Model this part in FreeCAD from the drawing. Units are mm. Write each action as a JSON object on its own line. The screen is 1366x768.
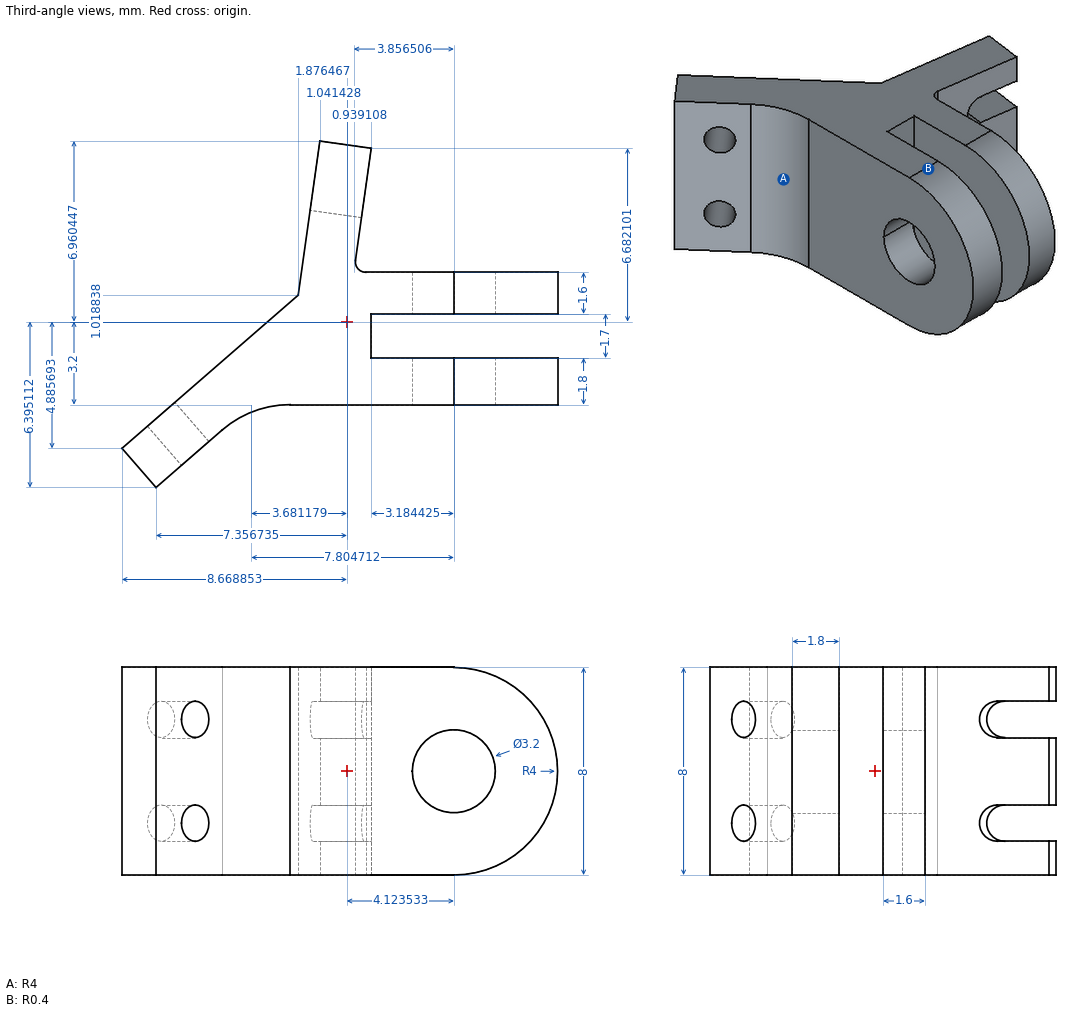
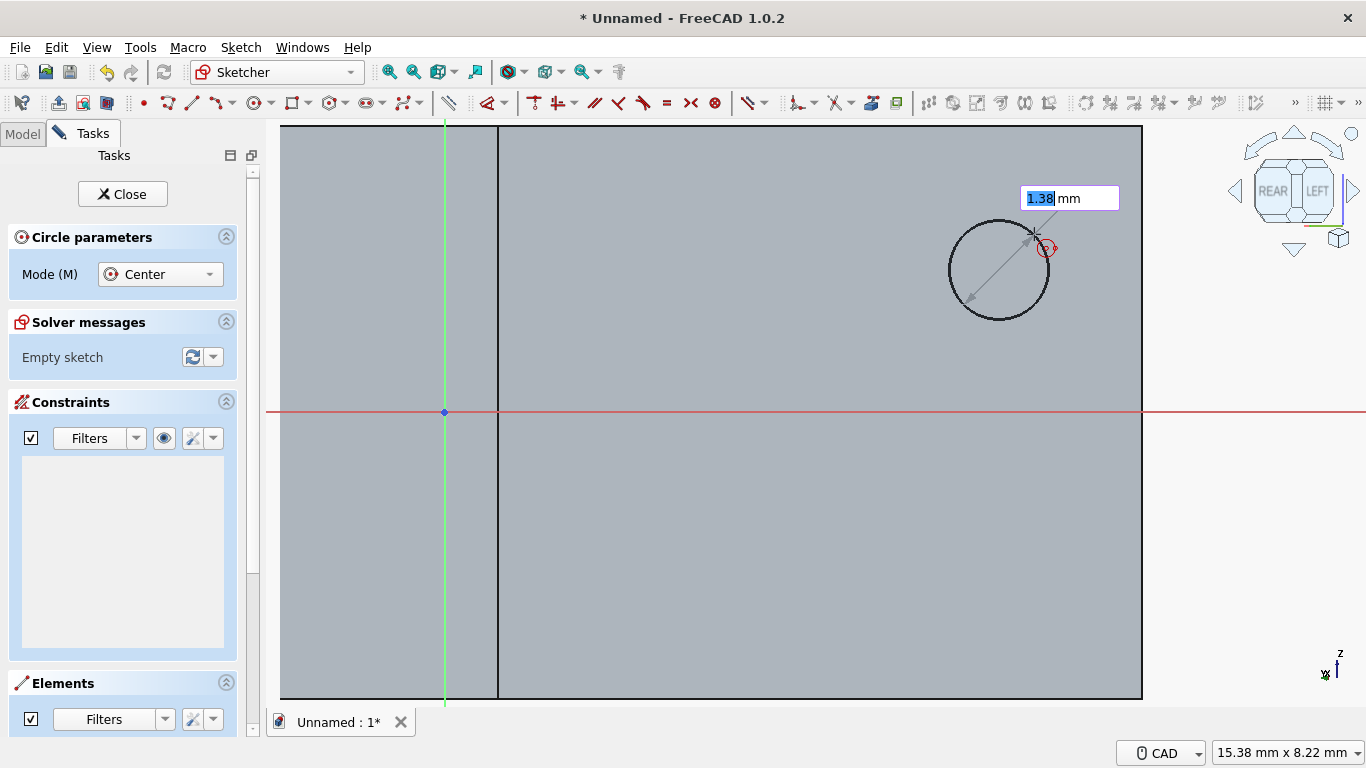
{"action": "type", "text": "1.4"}
{"action": "key", "text": "Return"}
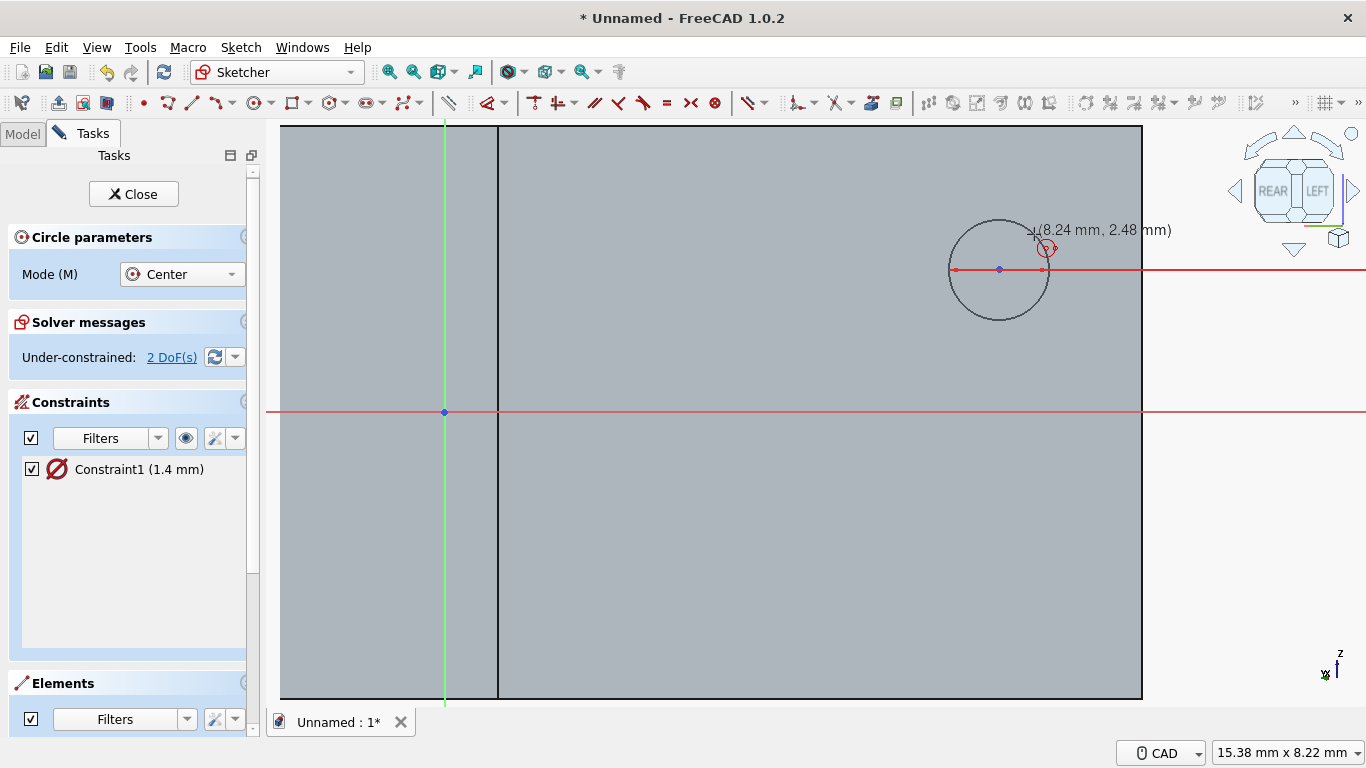
{"action": "left_click", "coordinate": [999, 555]}
{"action": "mouse_move", "coordinate": [1034, 520]}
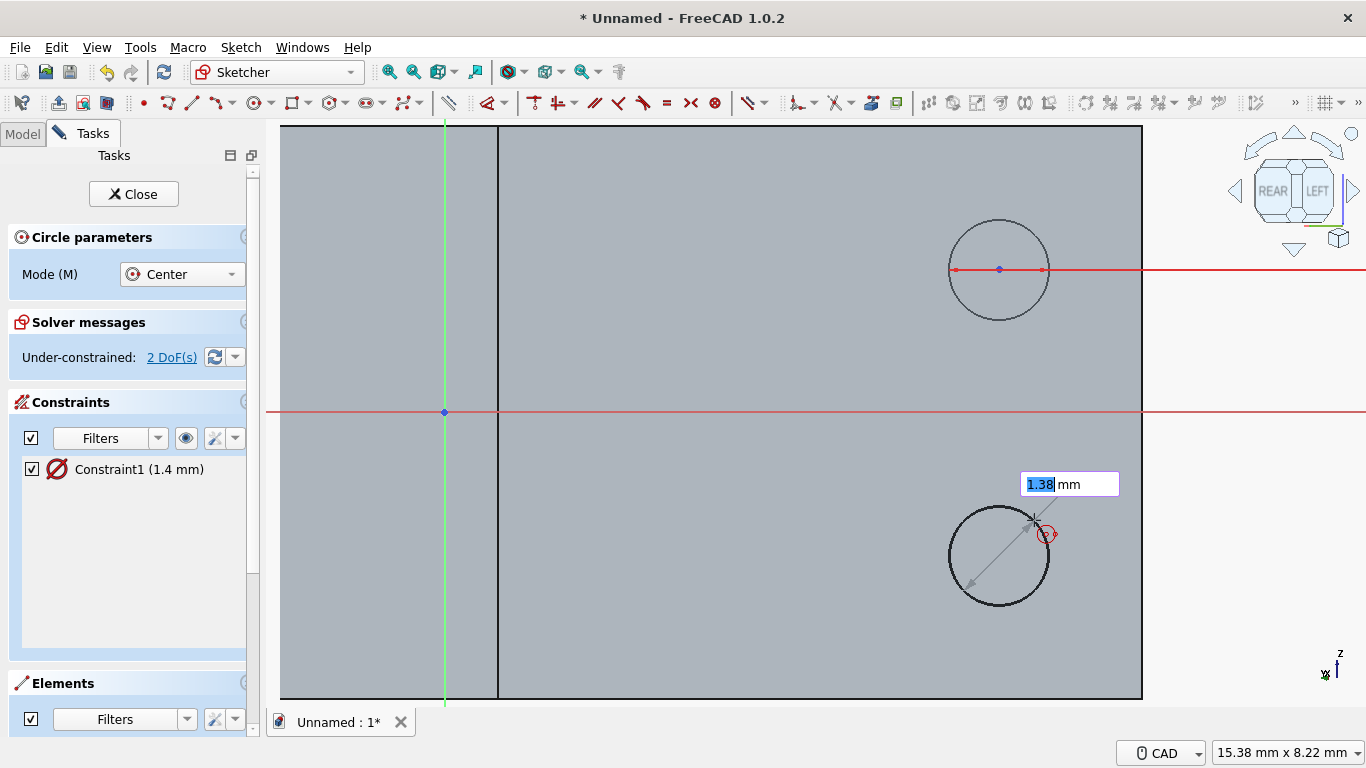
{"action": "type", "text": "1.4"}
{"action": "key", "text": "Return"}
{"action": "key", "text": "Escape"}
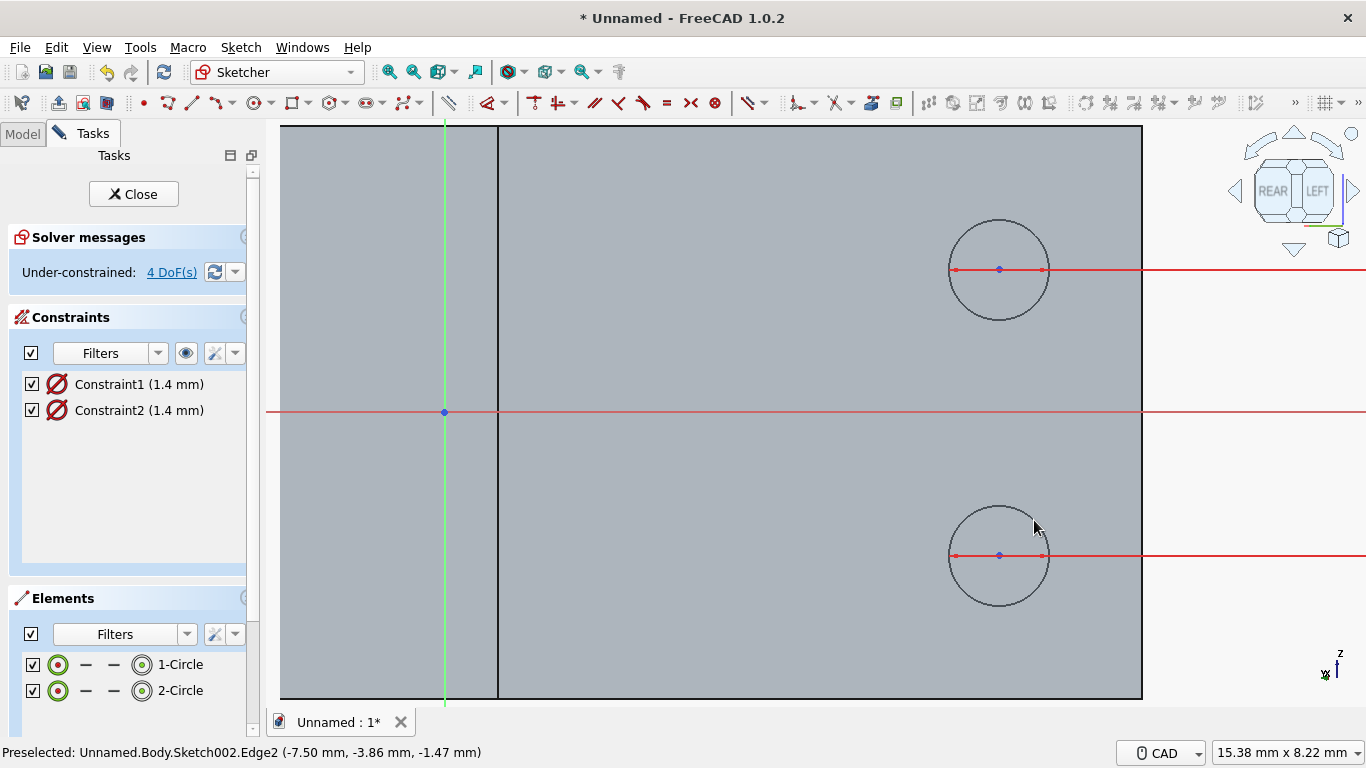
{"action": "left_click", "coordinate": [999, 270]}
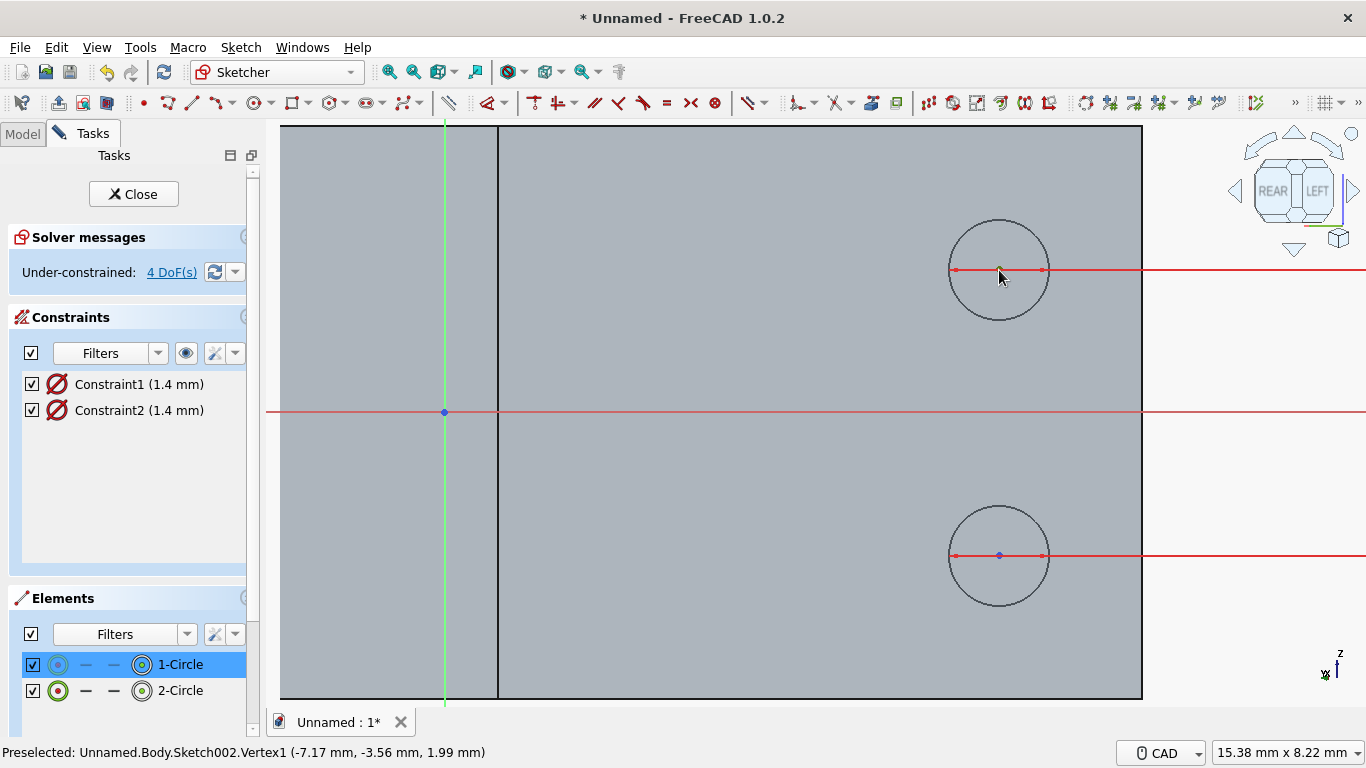
{"action": "left_click", "coordinate": [999, 556]}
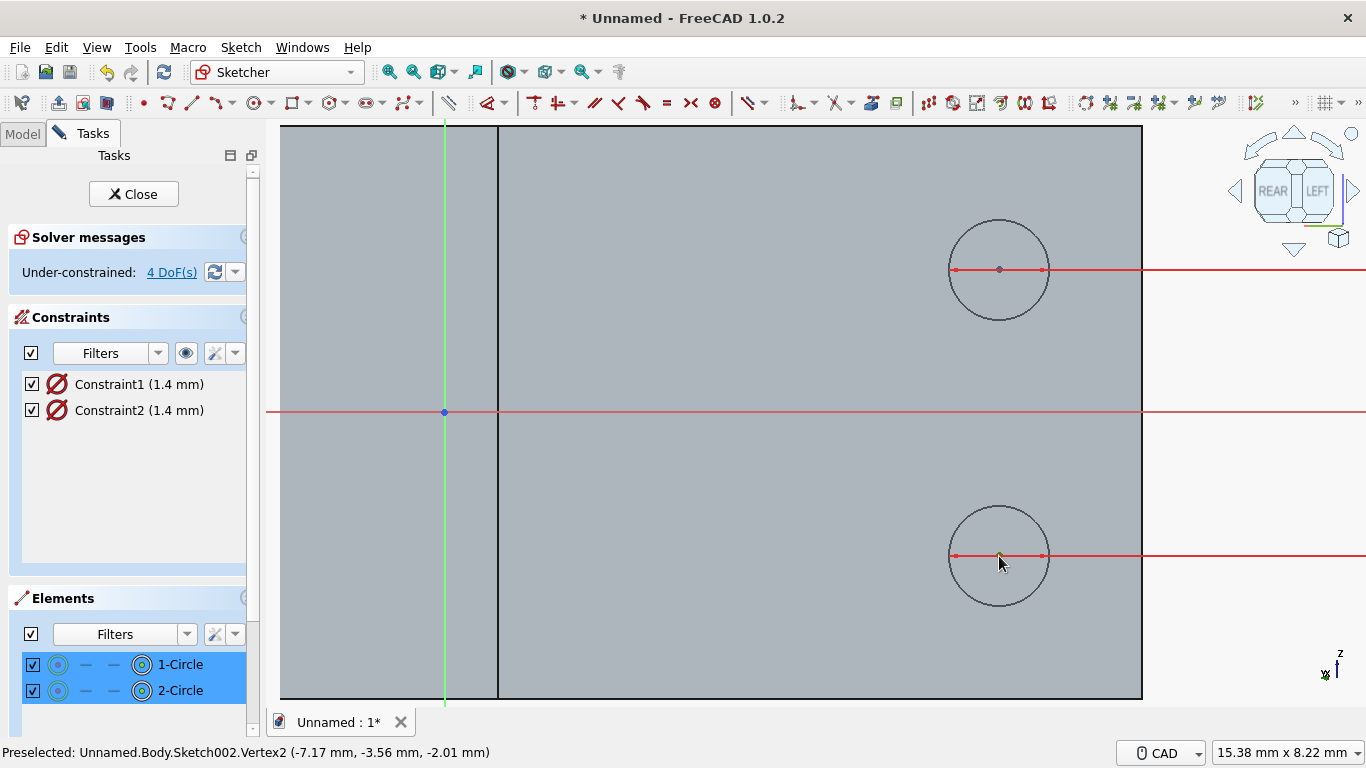
{"action": "left_click", "coordinate": [576, 104]}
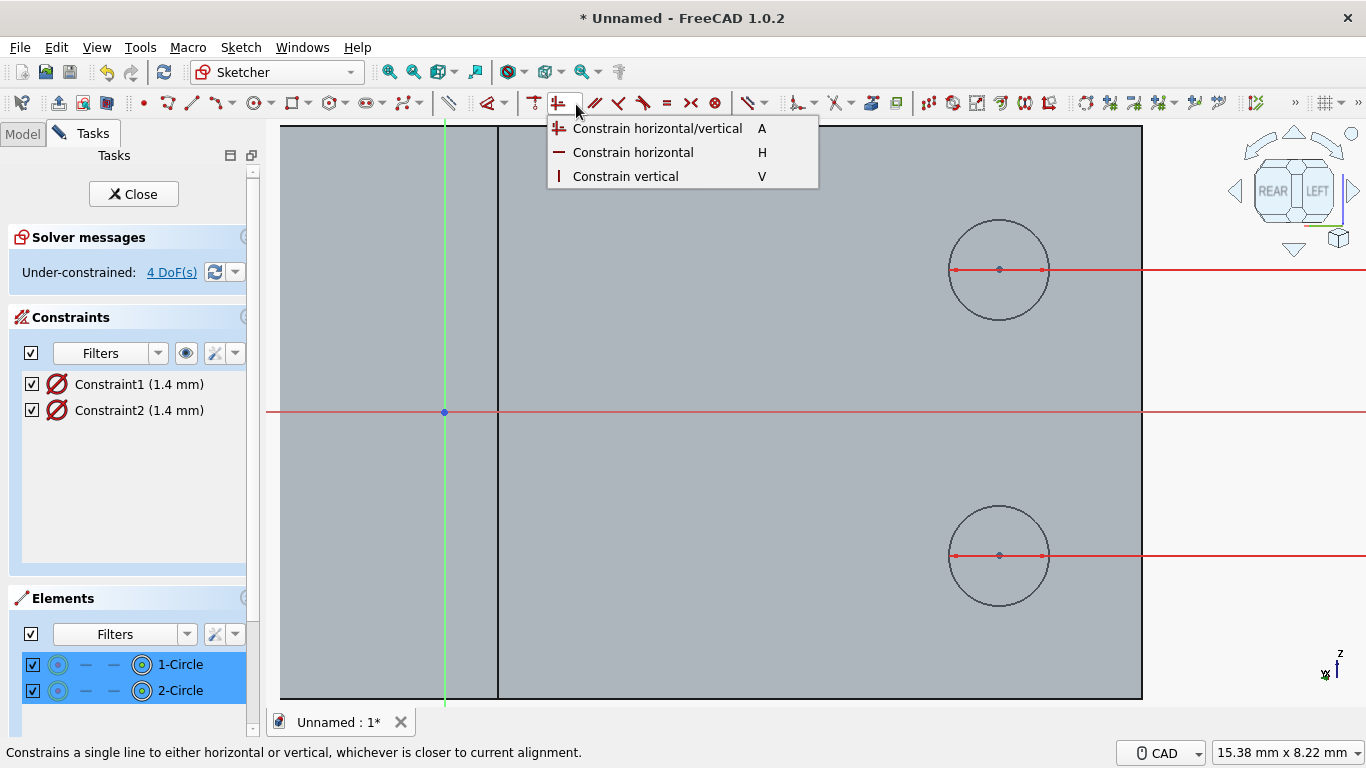
{"action": "left_click", "coordinate": [683, 176]}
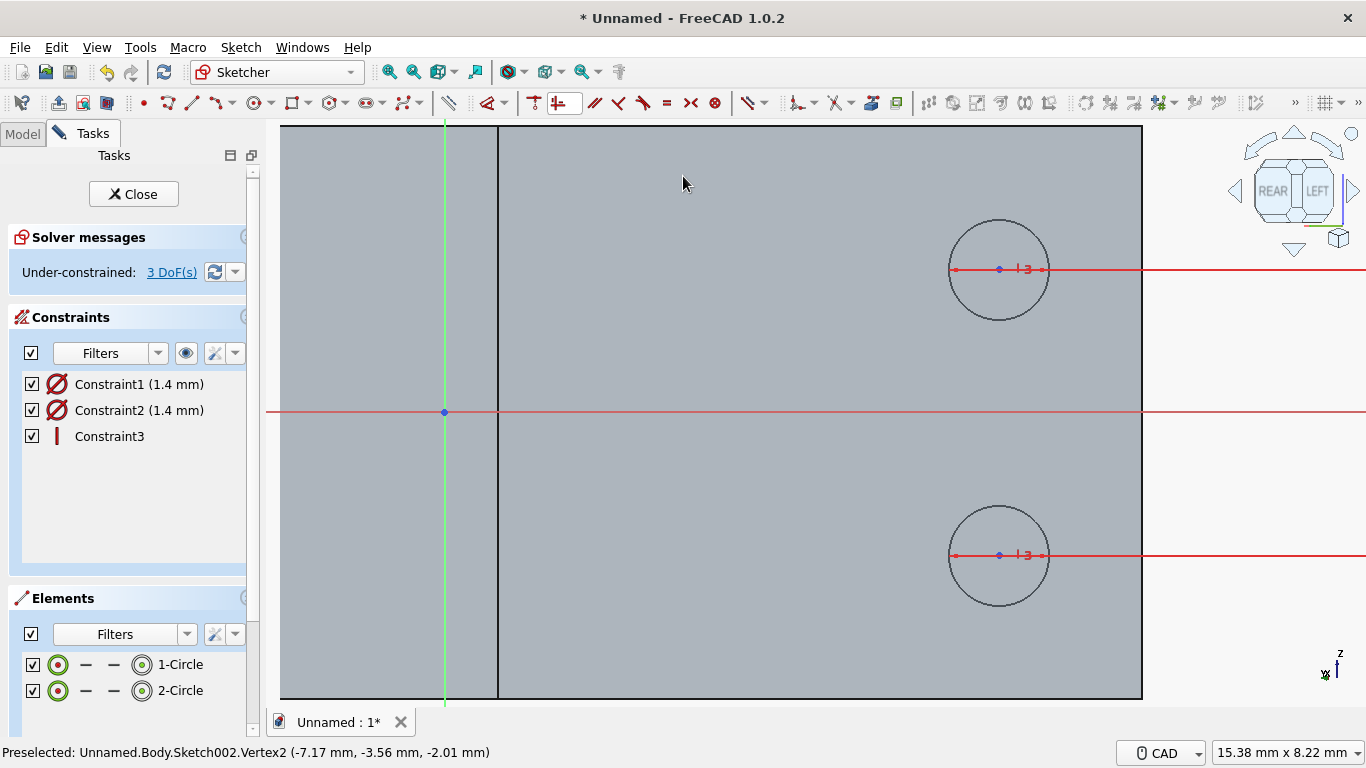
{"action": "left_click", "coordinate": [488, 104]}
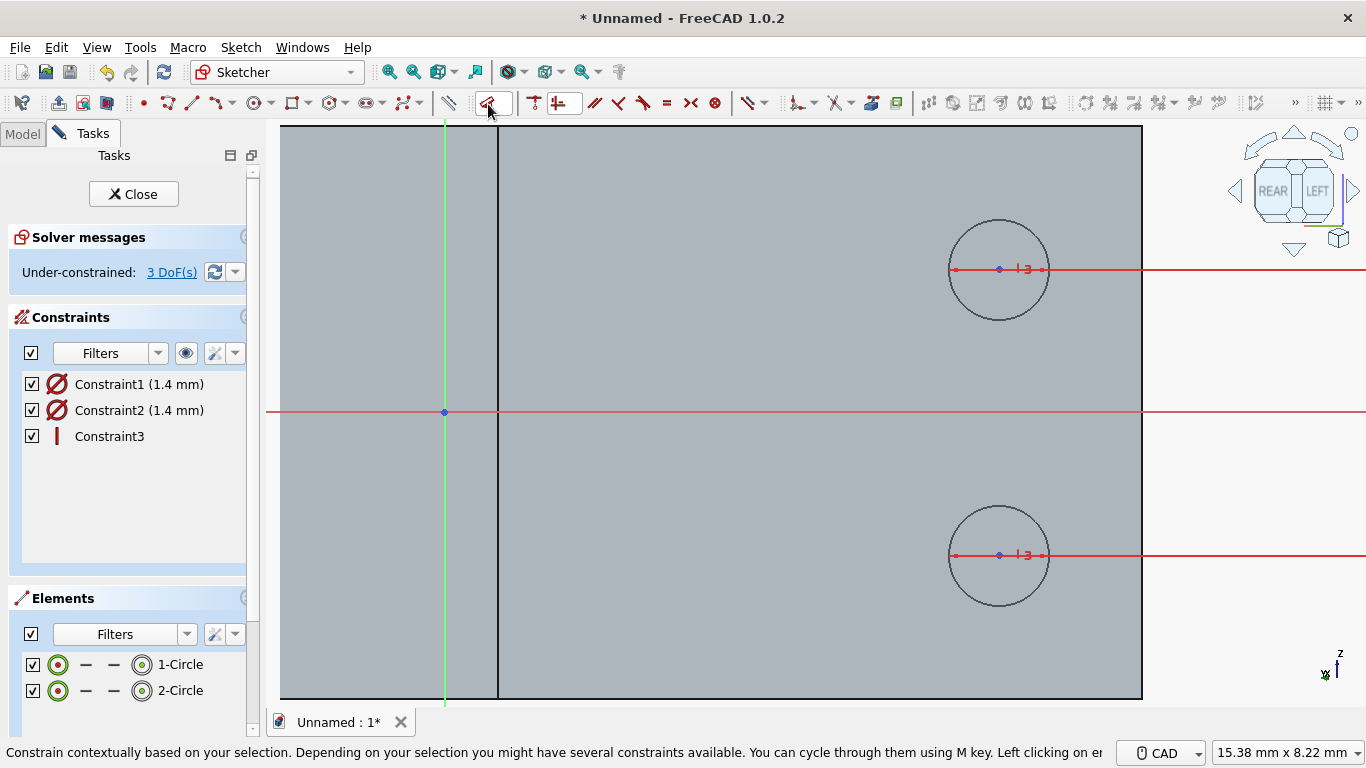
{"action": "left_click", "coordinate": [999, 270]}
{"action": "left_click", "coordinate": [411, 341]}